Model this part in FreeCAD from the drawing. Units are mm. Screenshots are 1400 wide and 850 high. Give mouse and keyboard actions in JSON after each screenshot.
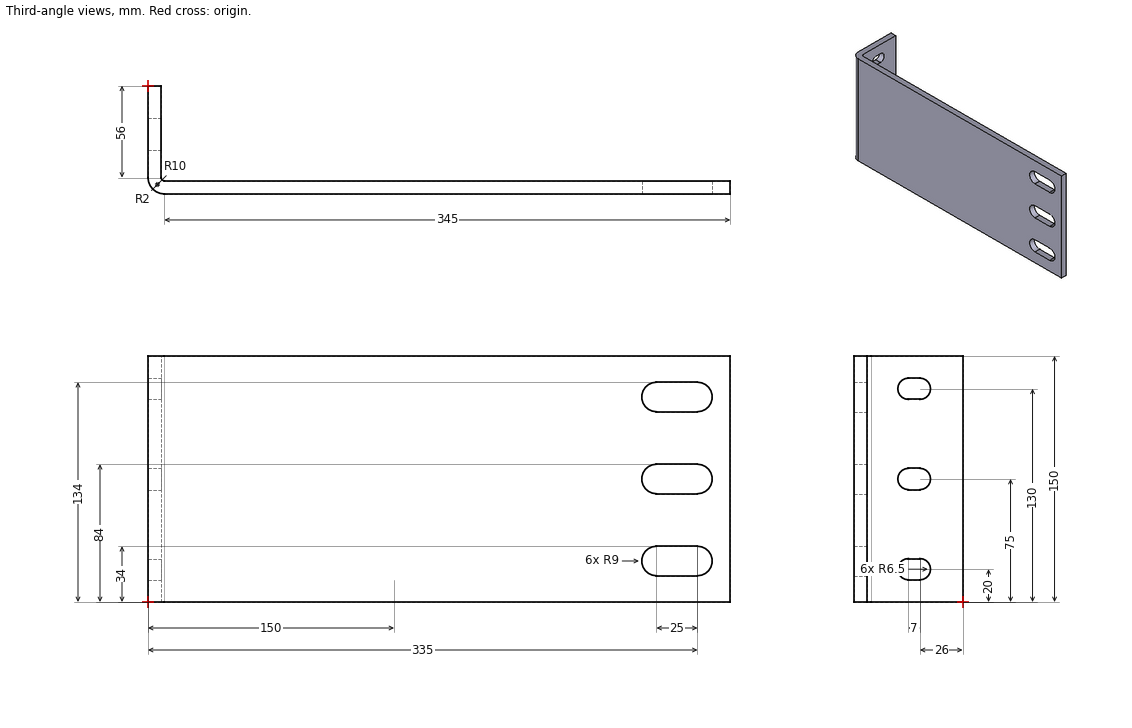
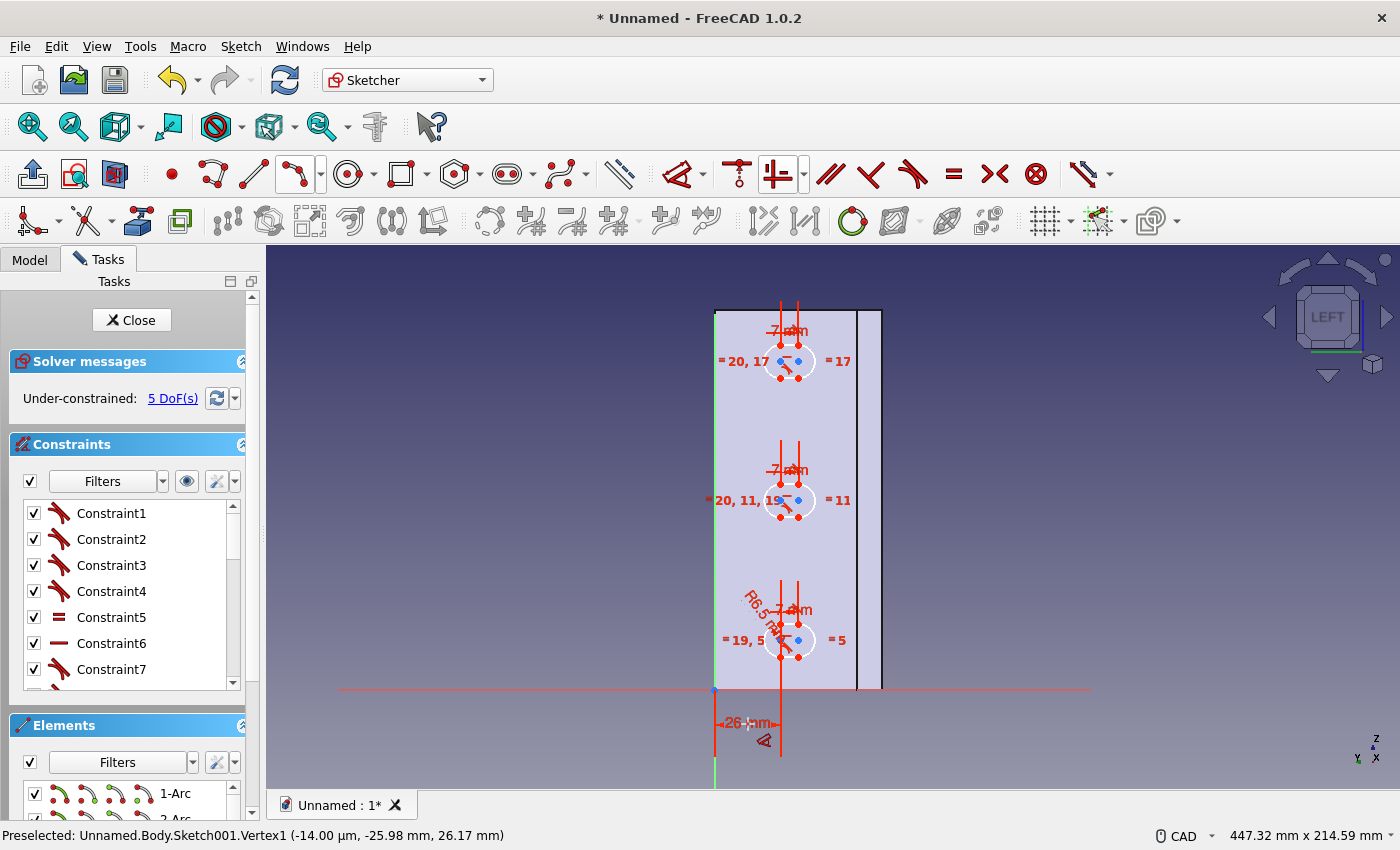
{"action": "left_click", "coordinate": [781, 484]}
{"action": "left_click", "coordinate": [748, 450]}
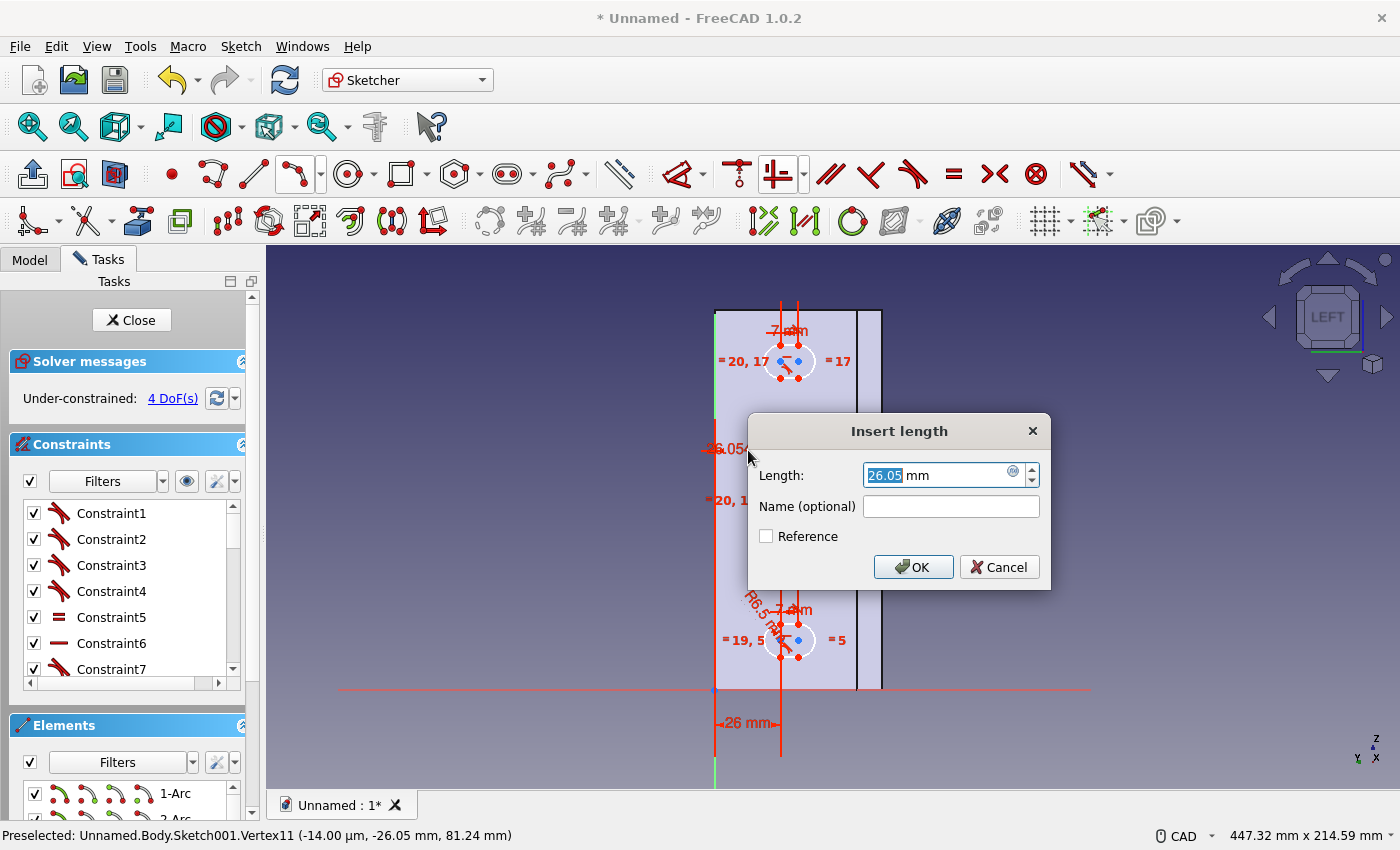
{"action": "type", "text": "26"}
{"action": "key", "text": "Return"}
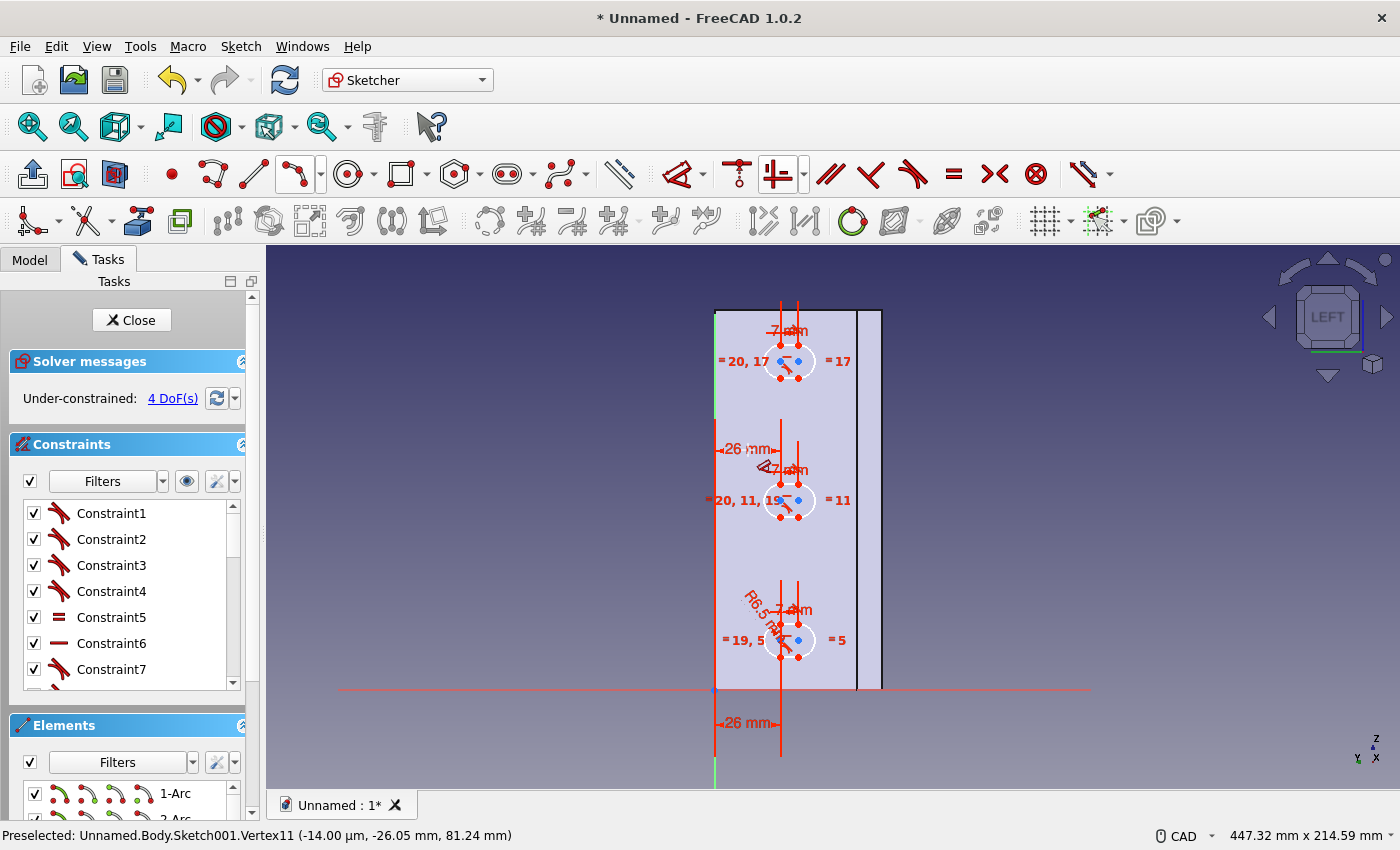
{"action": "left_click", "coordinate": [781, 345]}
{"action": "left_click", "coordinate": [748, 311]}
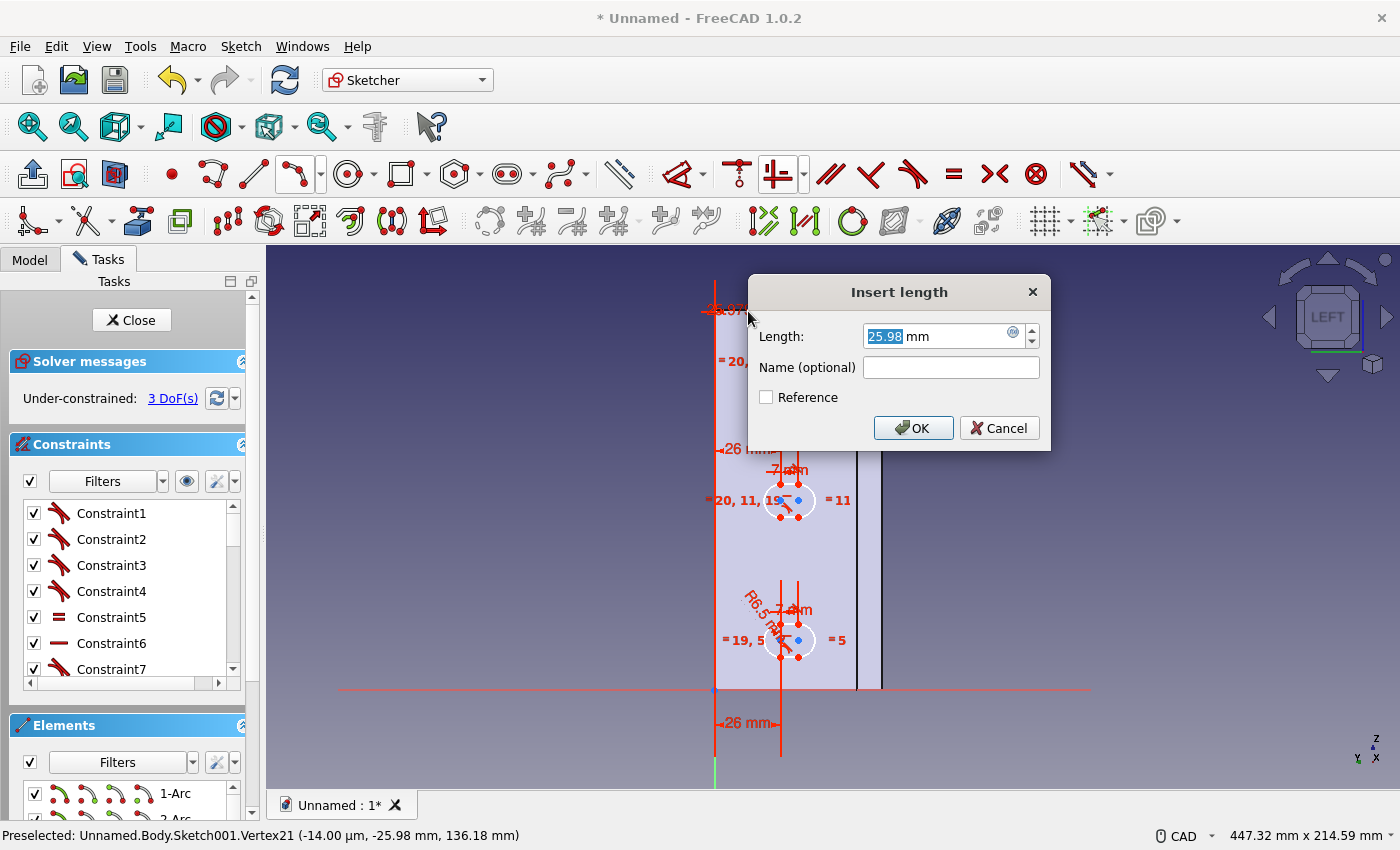
{"action": "type", "text": "26"}
{"action": "key", "text": "Return"}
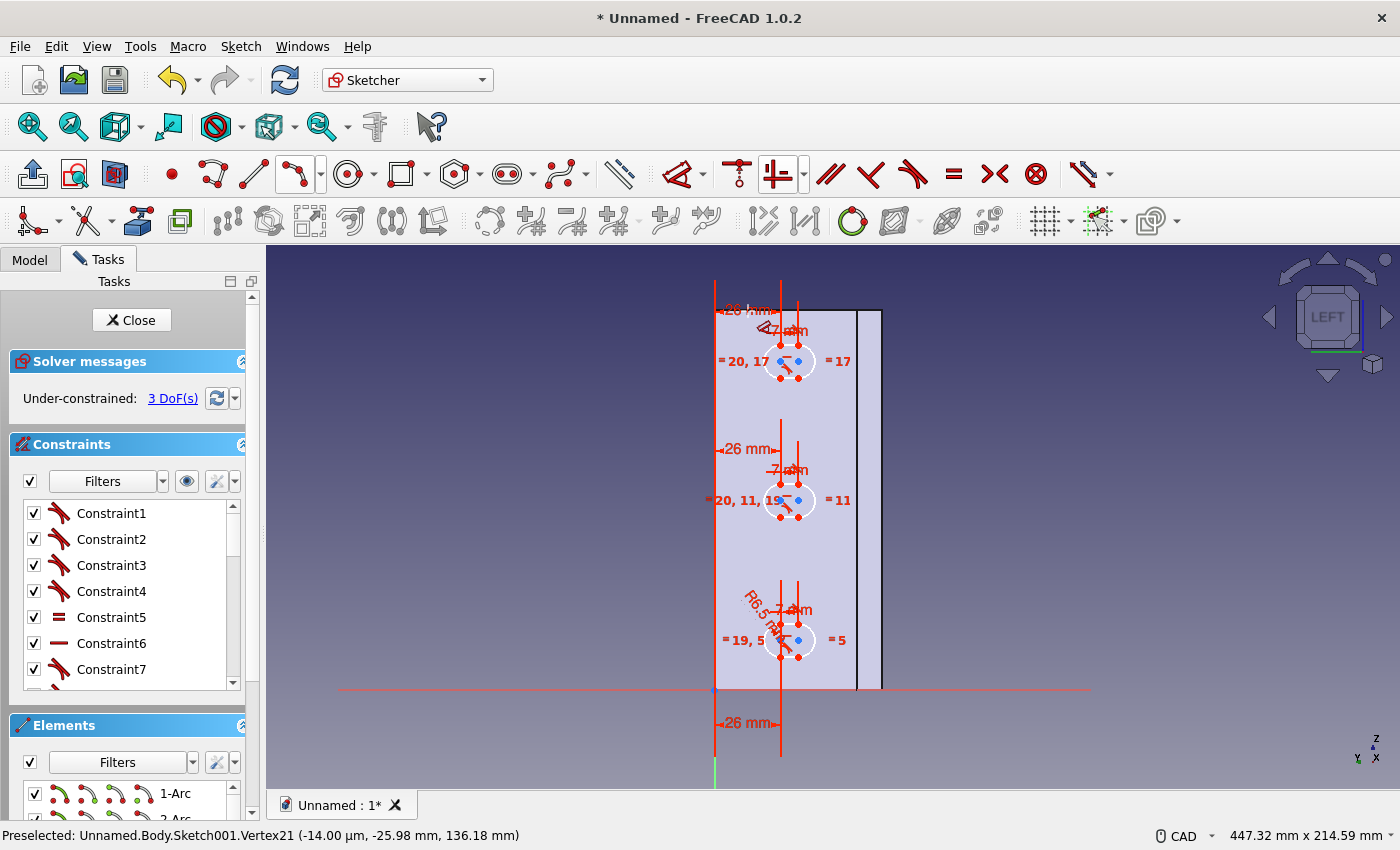
{"action": "left_click", "coordinate": [781, 641]}
{"action": "left_click", "coordinate": [681, 666]}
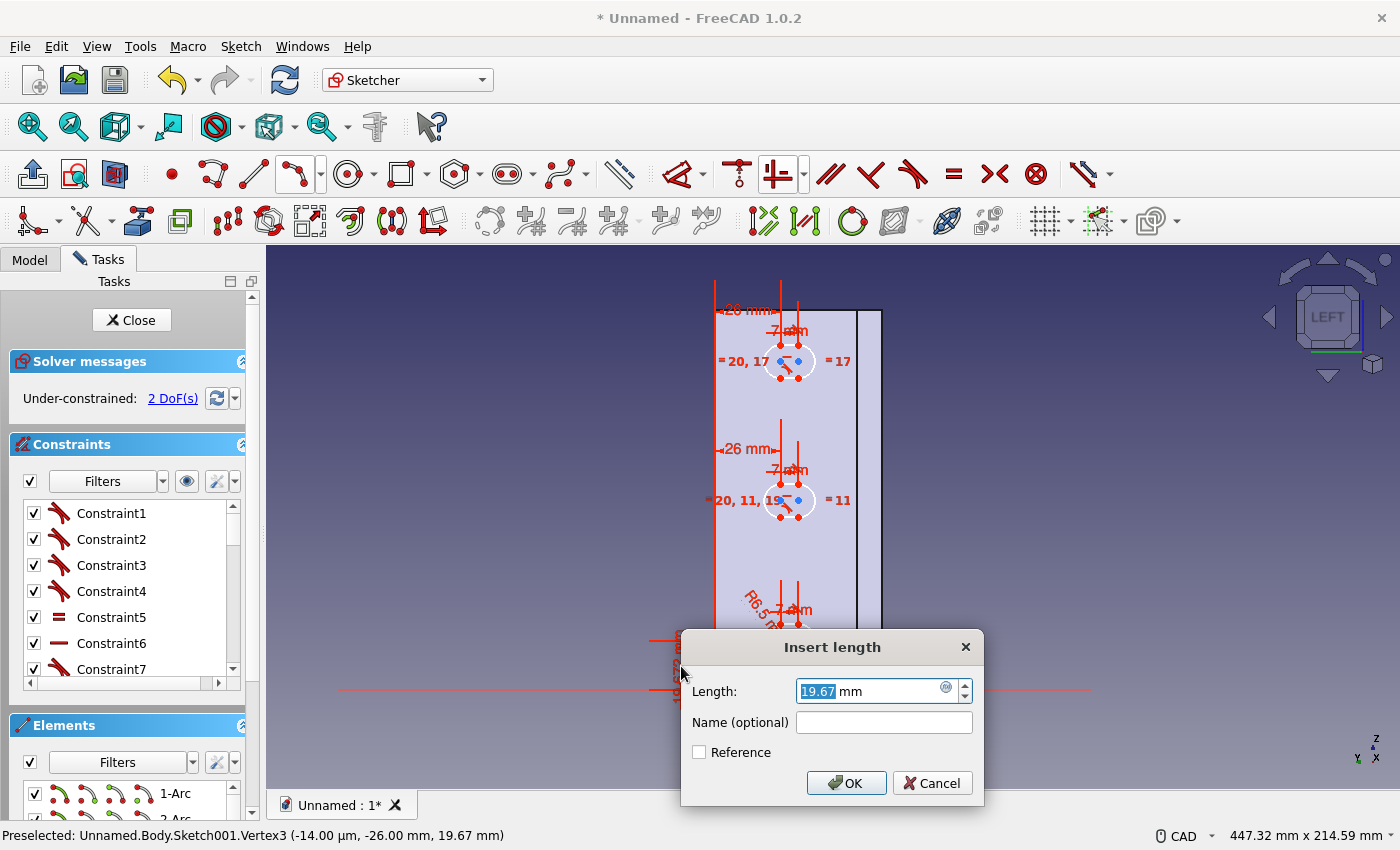
{"action": "type", "text": "20"}
{"action": "key", "text": "Return"}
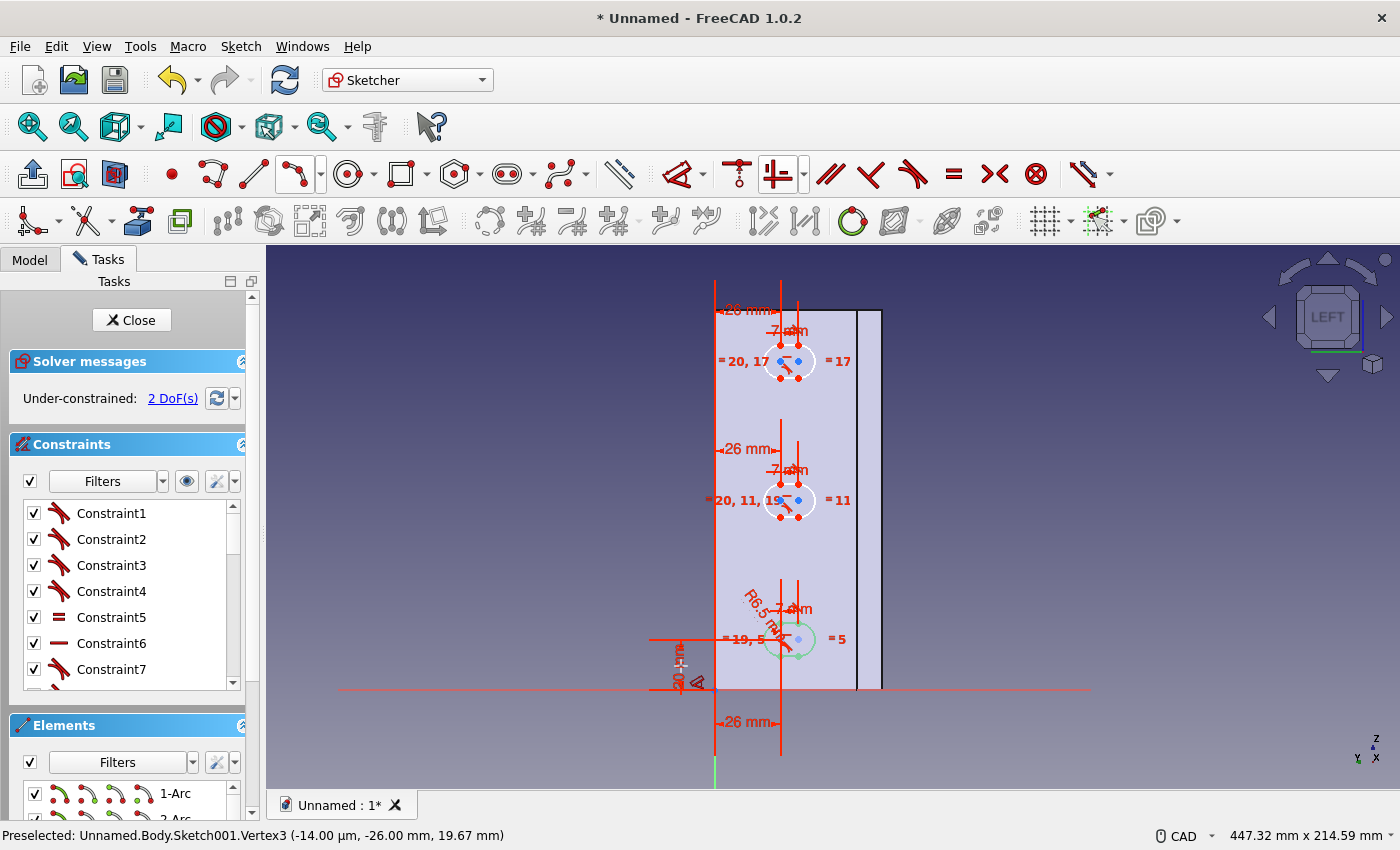
{"action": "left_click", "coordinate": [781, 501]}
{"action": "left_click", "coordinate": [681, 596]}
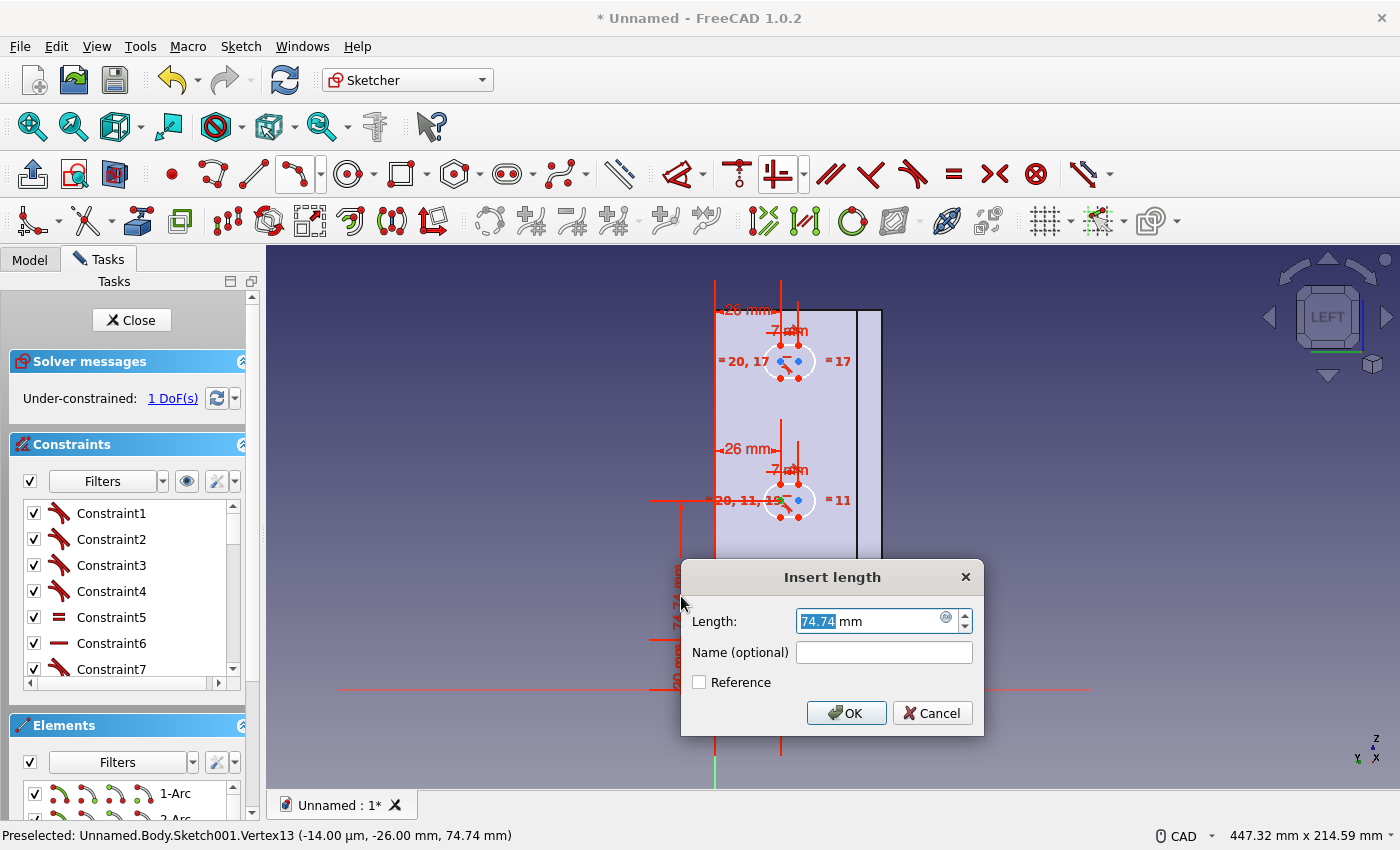
{"action": "type", "text": "75"}
{"action": "key", "text": "Return"}